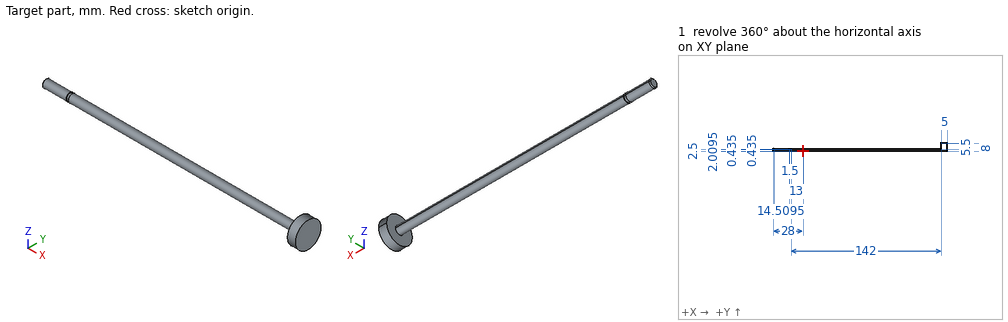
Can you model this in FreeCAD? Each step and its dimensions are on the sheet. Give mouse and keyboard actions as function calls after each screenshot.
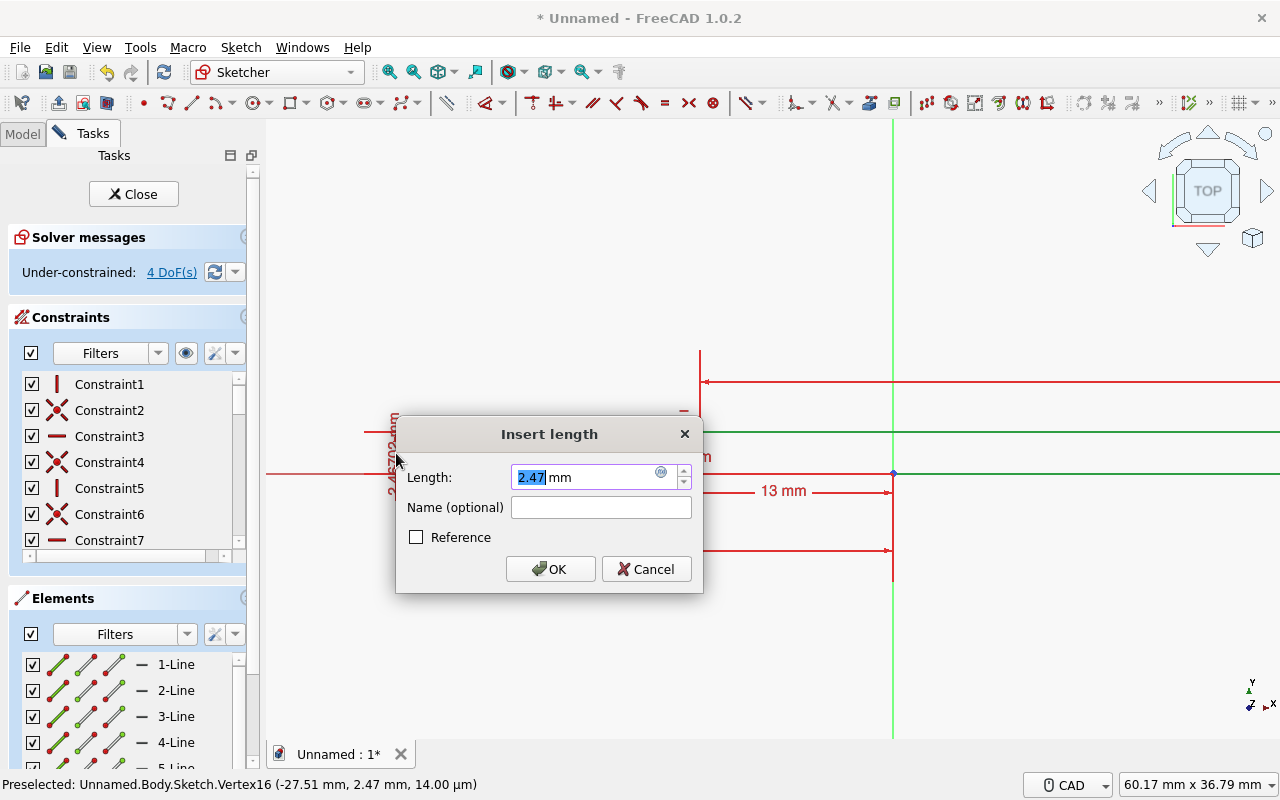
text(2.5)
key(Return)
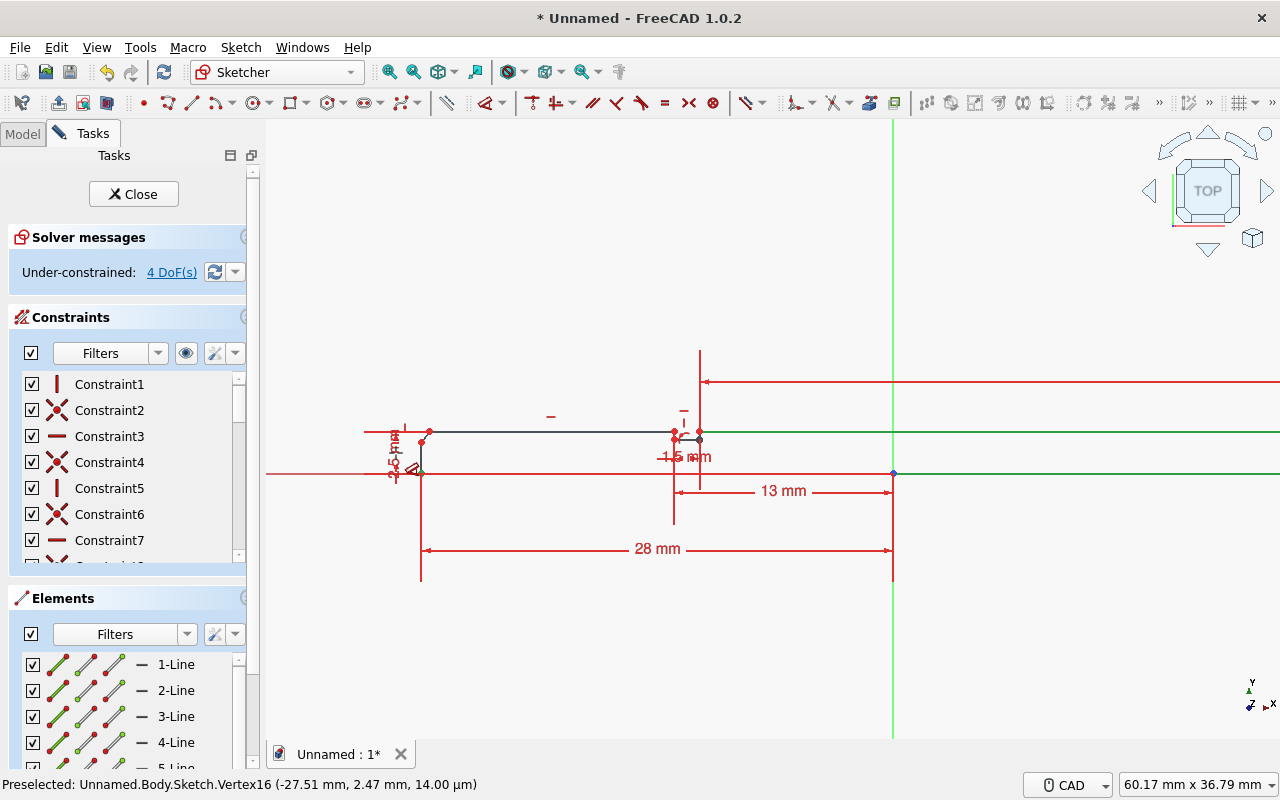
scroll(700, 436, up, 9)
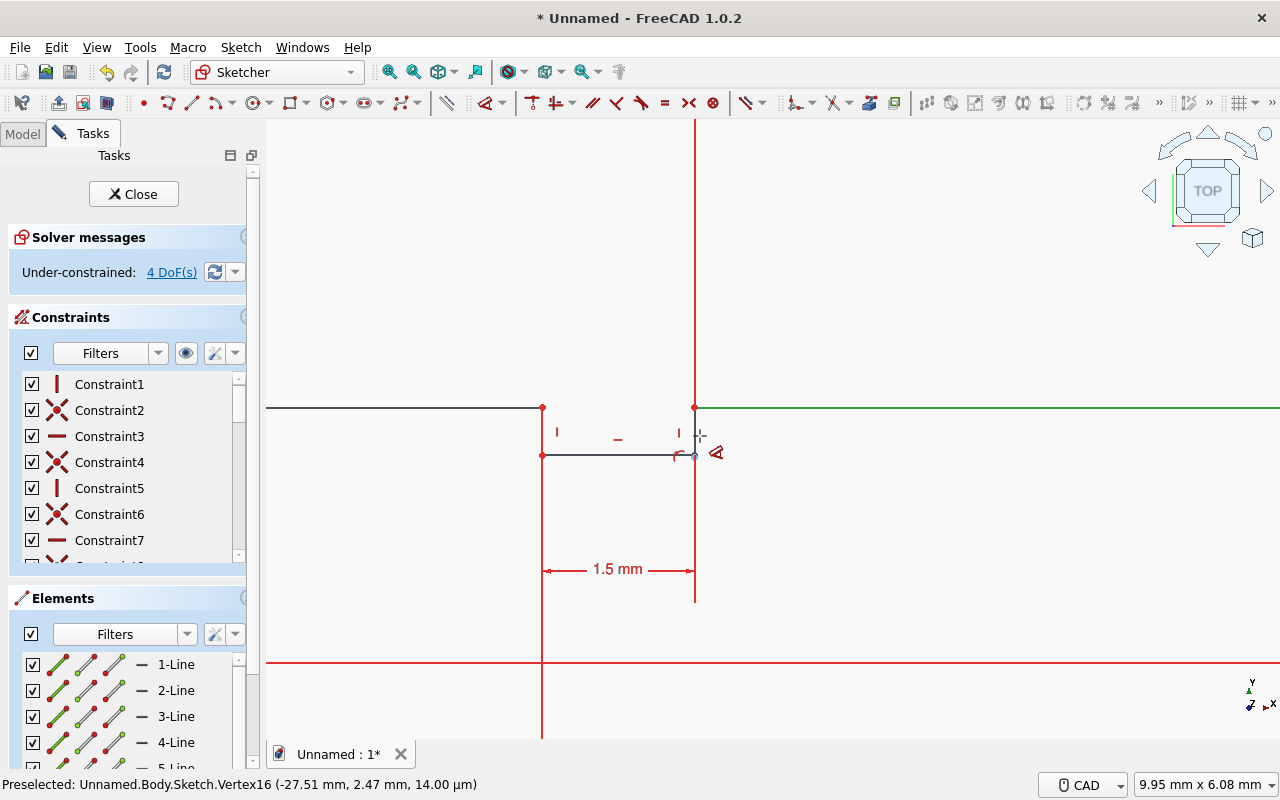
click(695, 433)
click(661, 433)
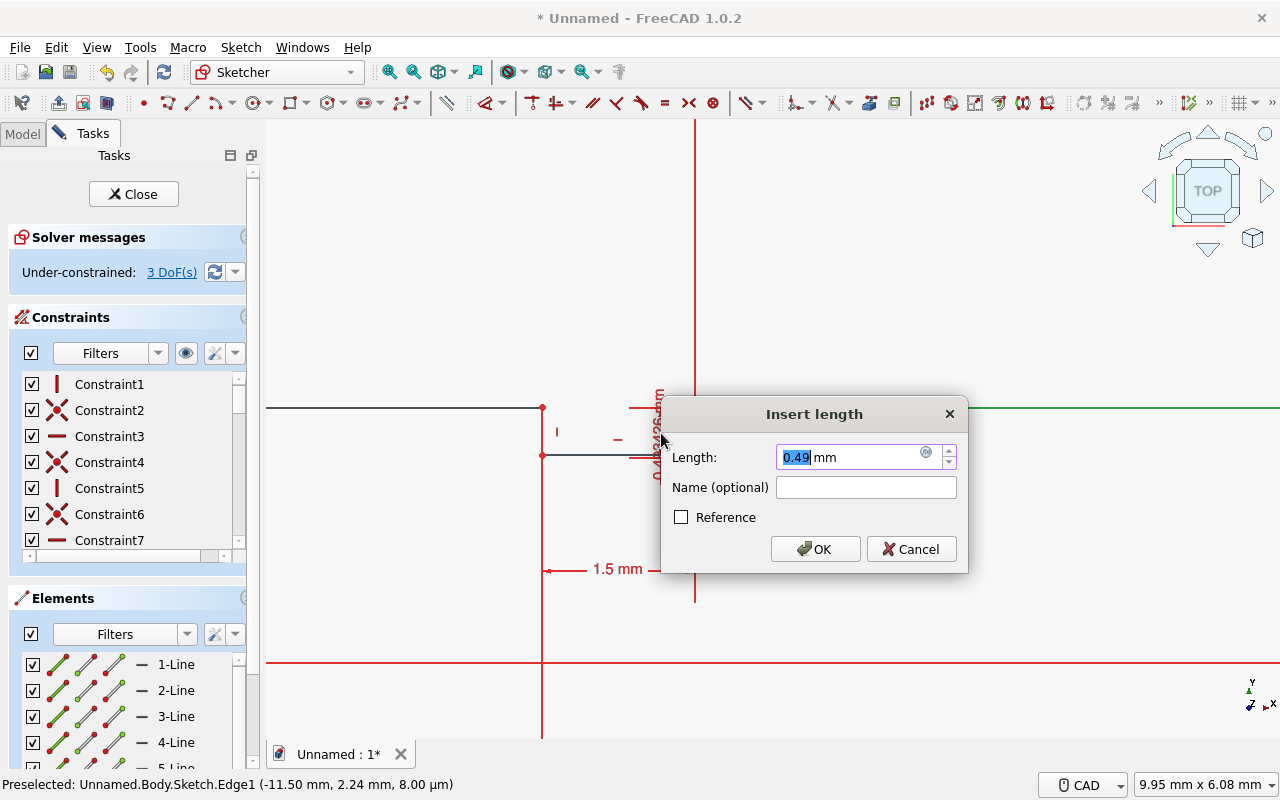
text(0.435)
key(Return)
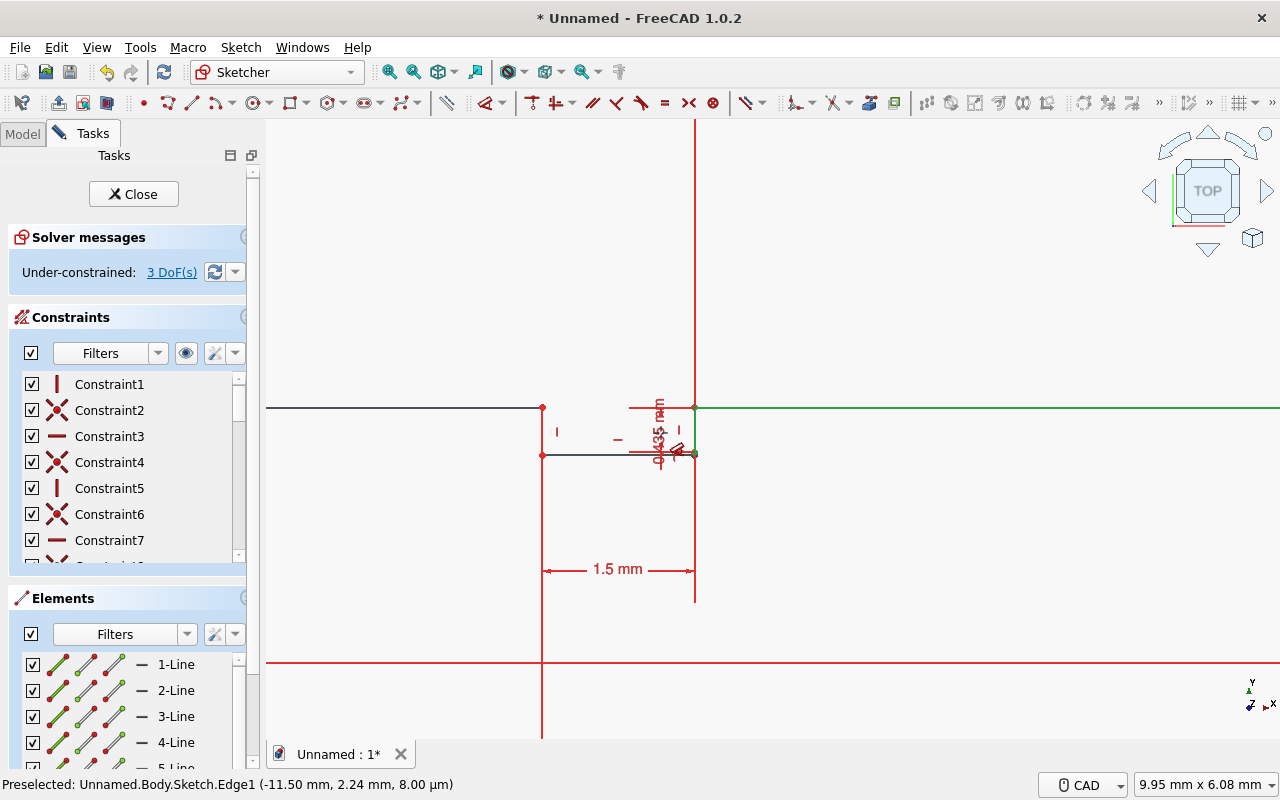
click(542, 422)
click(508, 431)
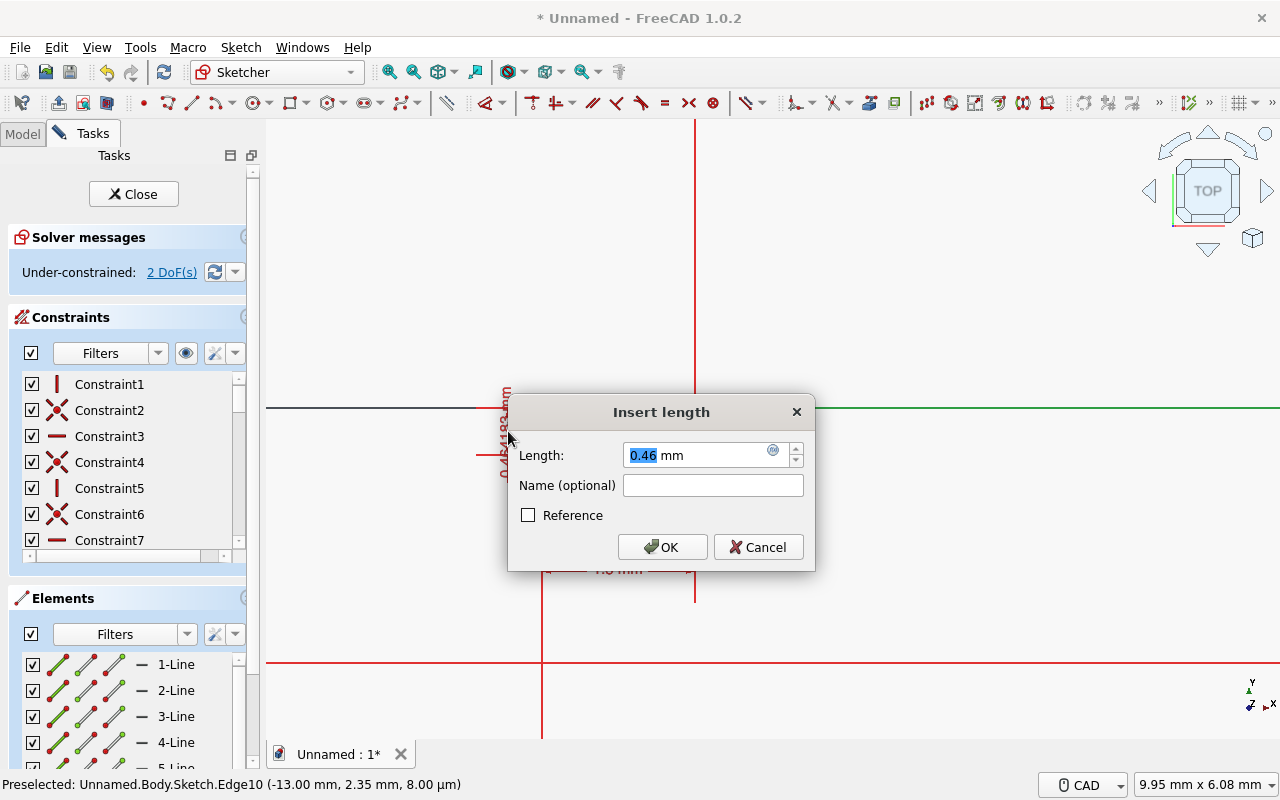
text(0.435)
key(Return)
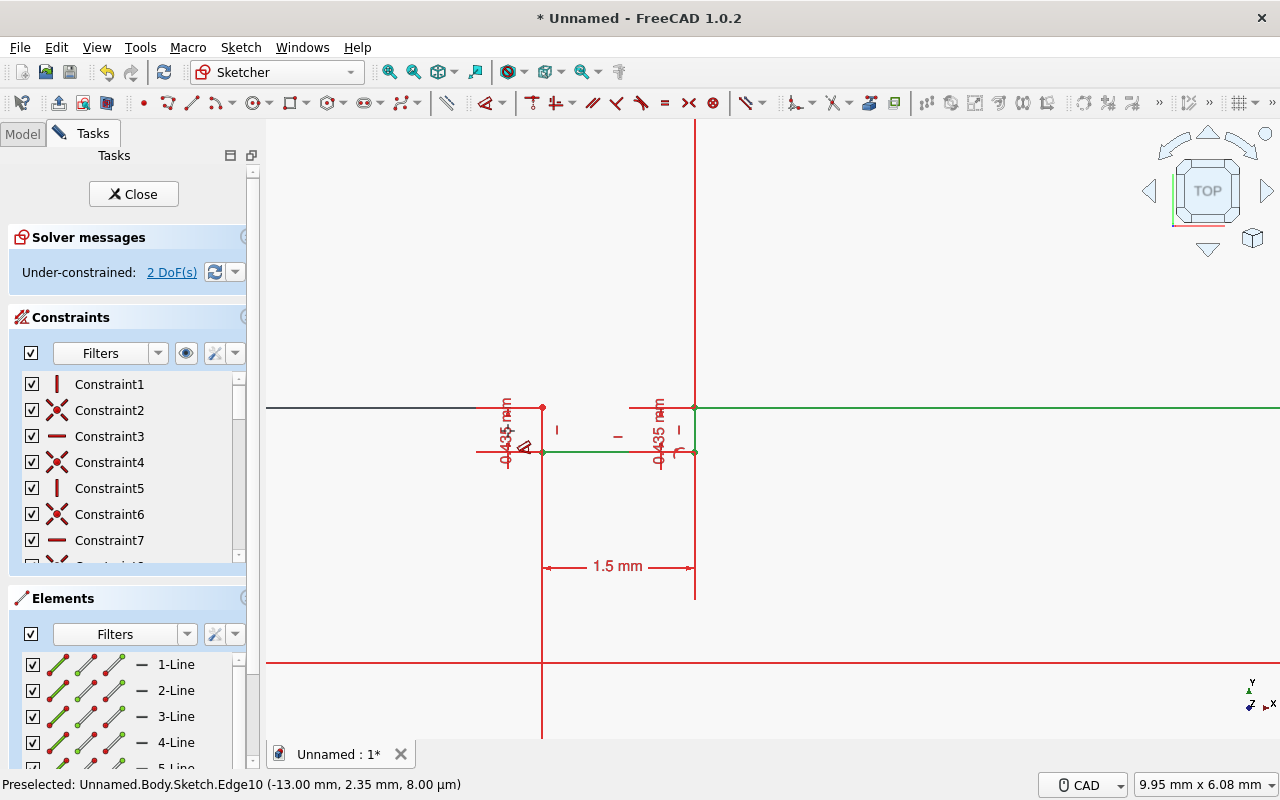
scroll(422, 436, down, 16)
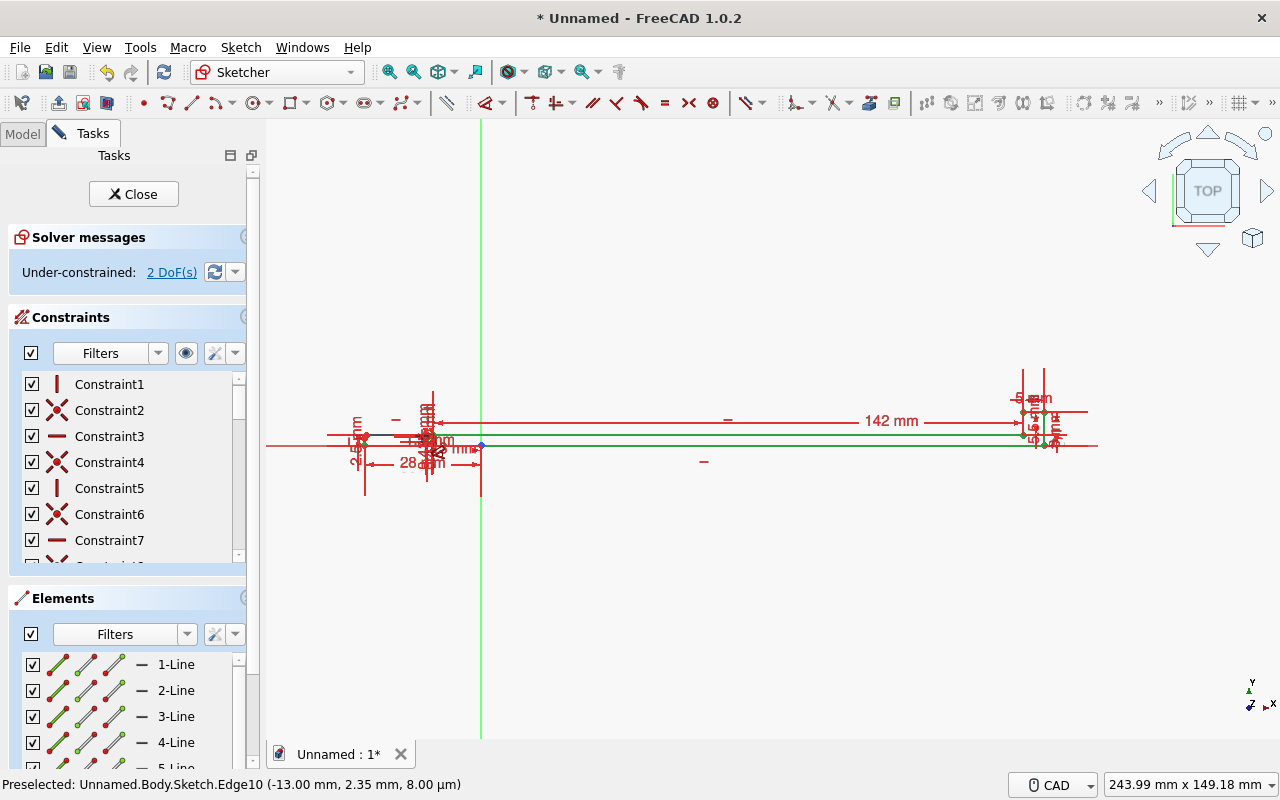
scroll(365, 443, up, 9)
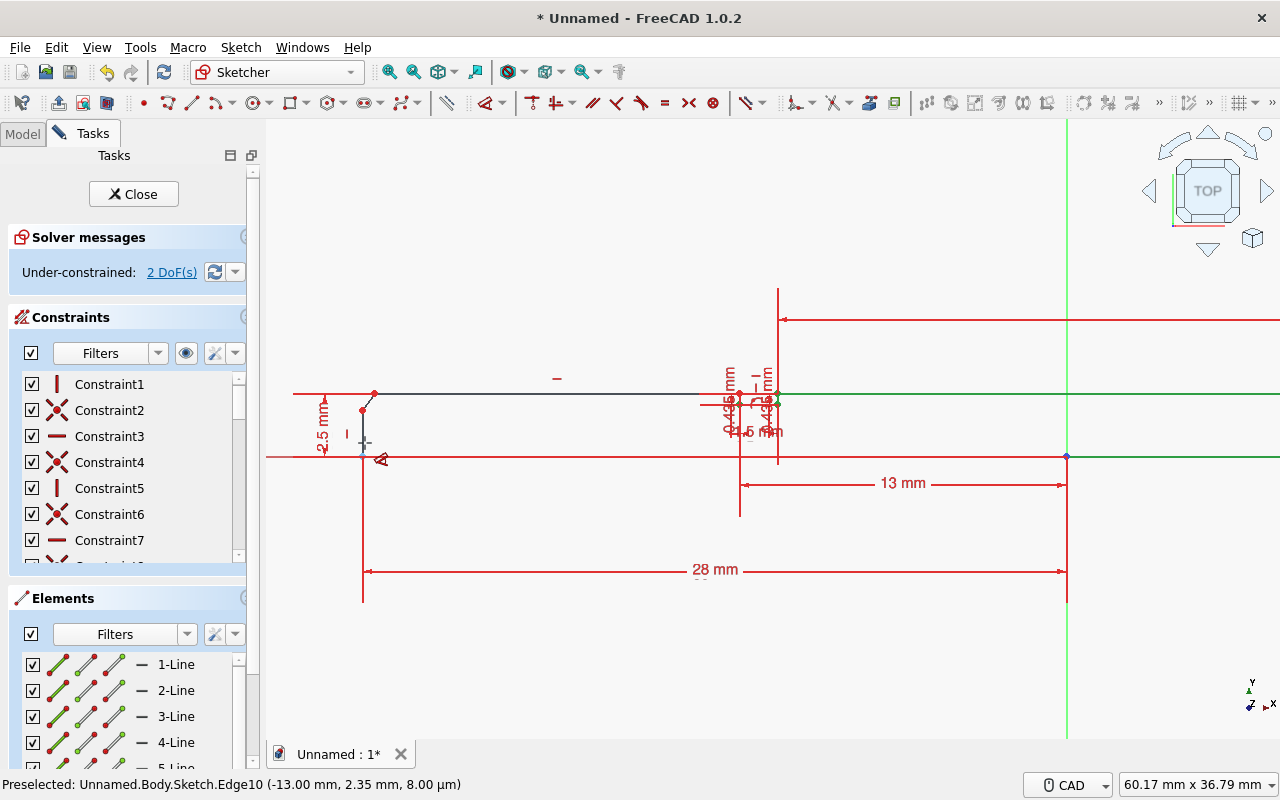
click(363, 443)
click(397, 434)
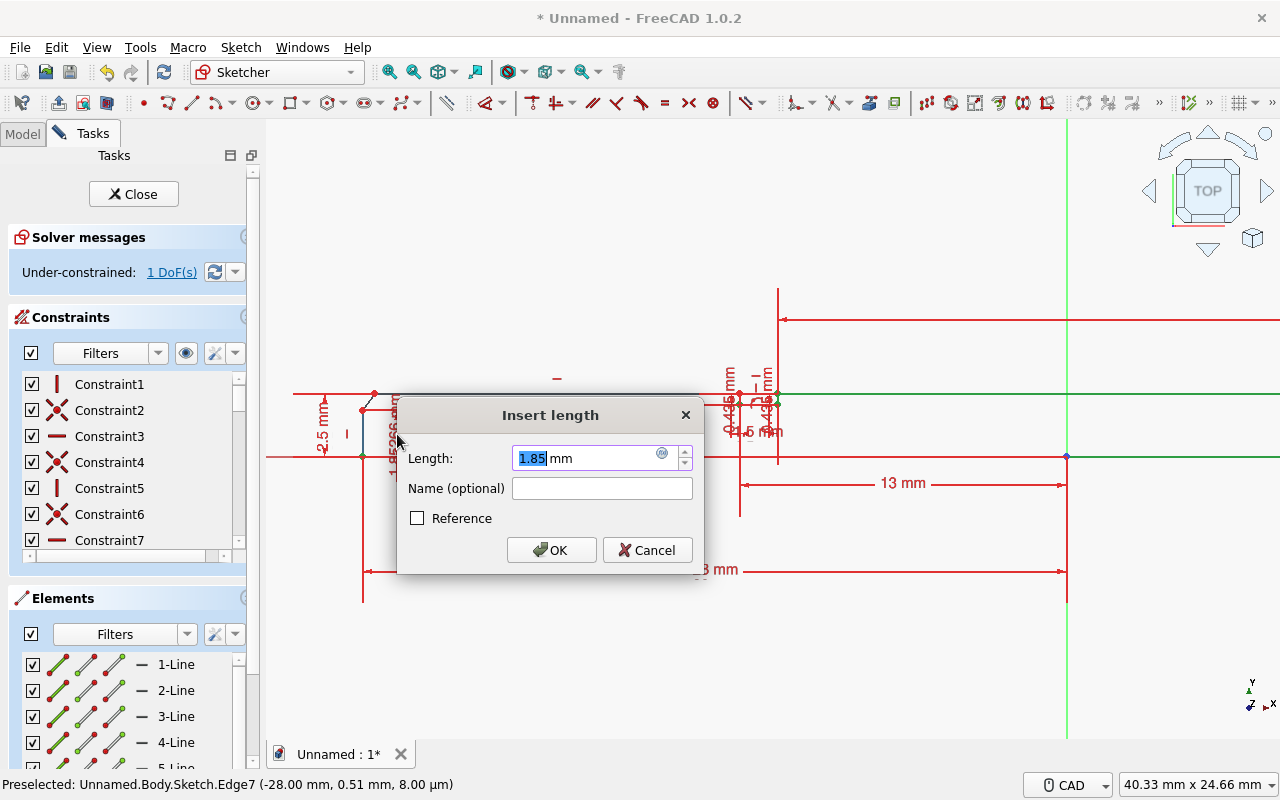
text(2.0095)
key(Return)